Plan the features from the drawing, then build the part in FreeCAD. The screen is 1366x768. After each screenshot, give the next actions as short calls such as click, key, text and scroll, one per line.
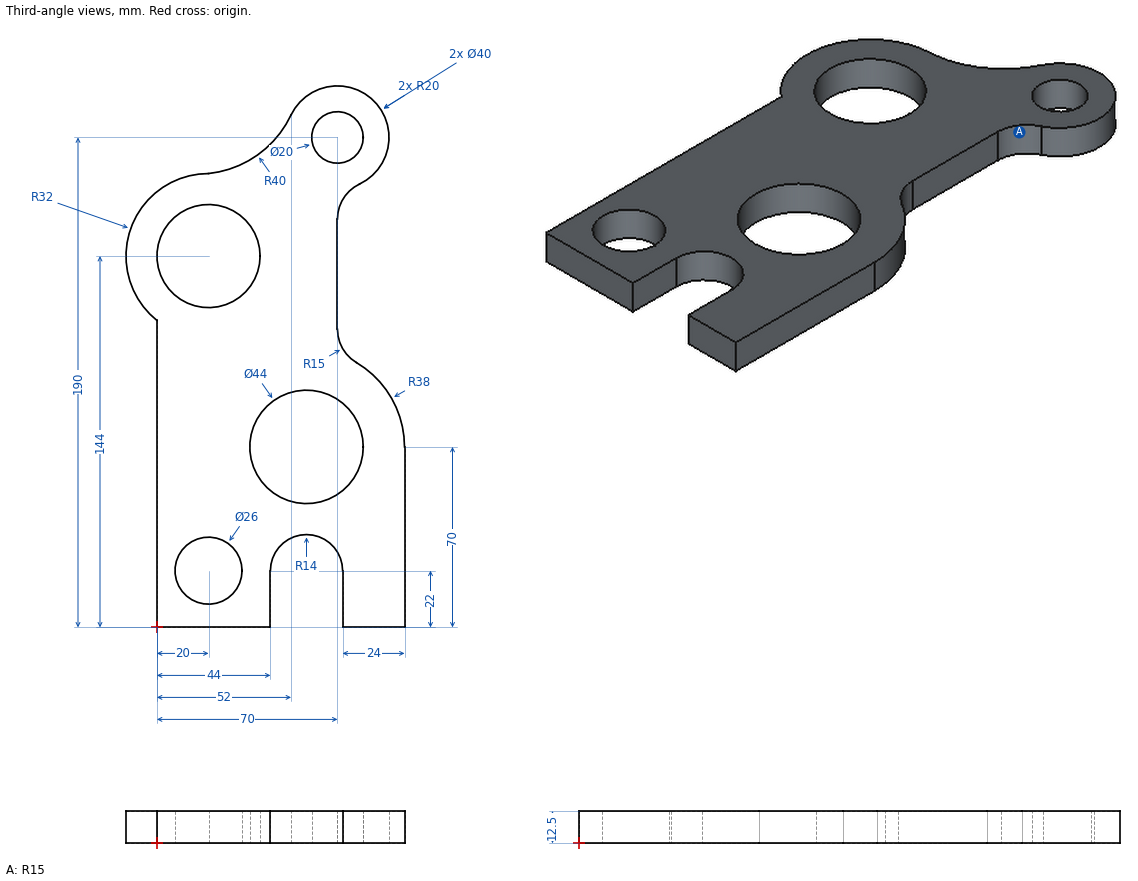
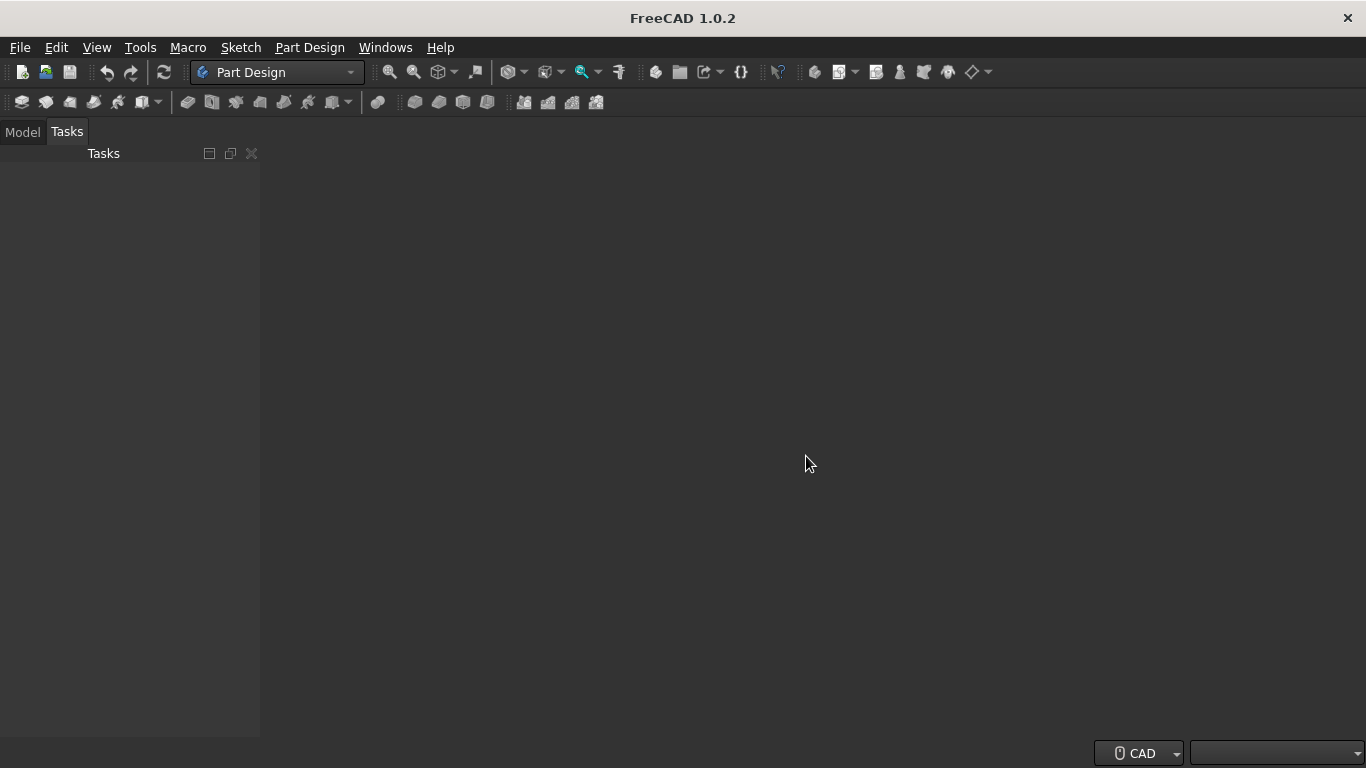
click(22, 72)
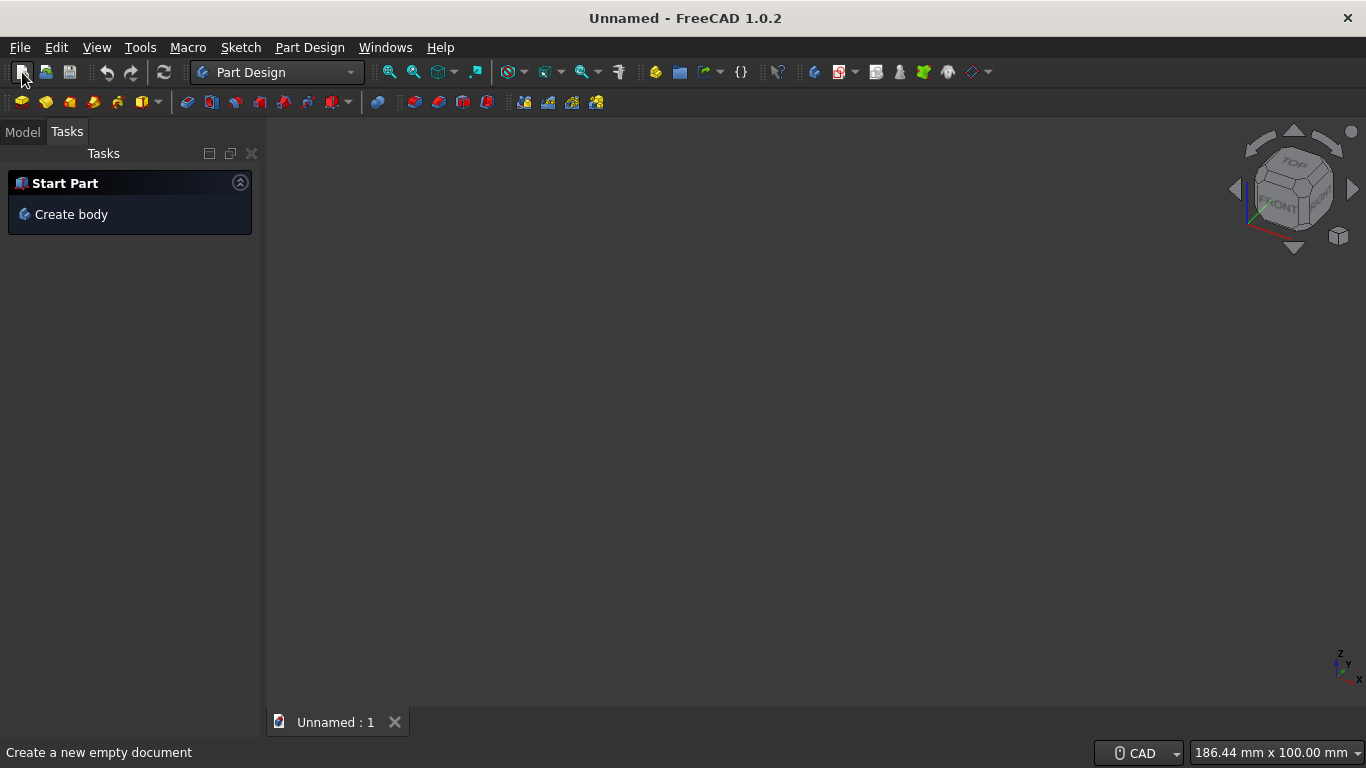
click(840, 72)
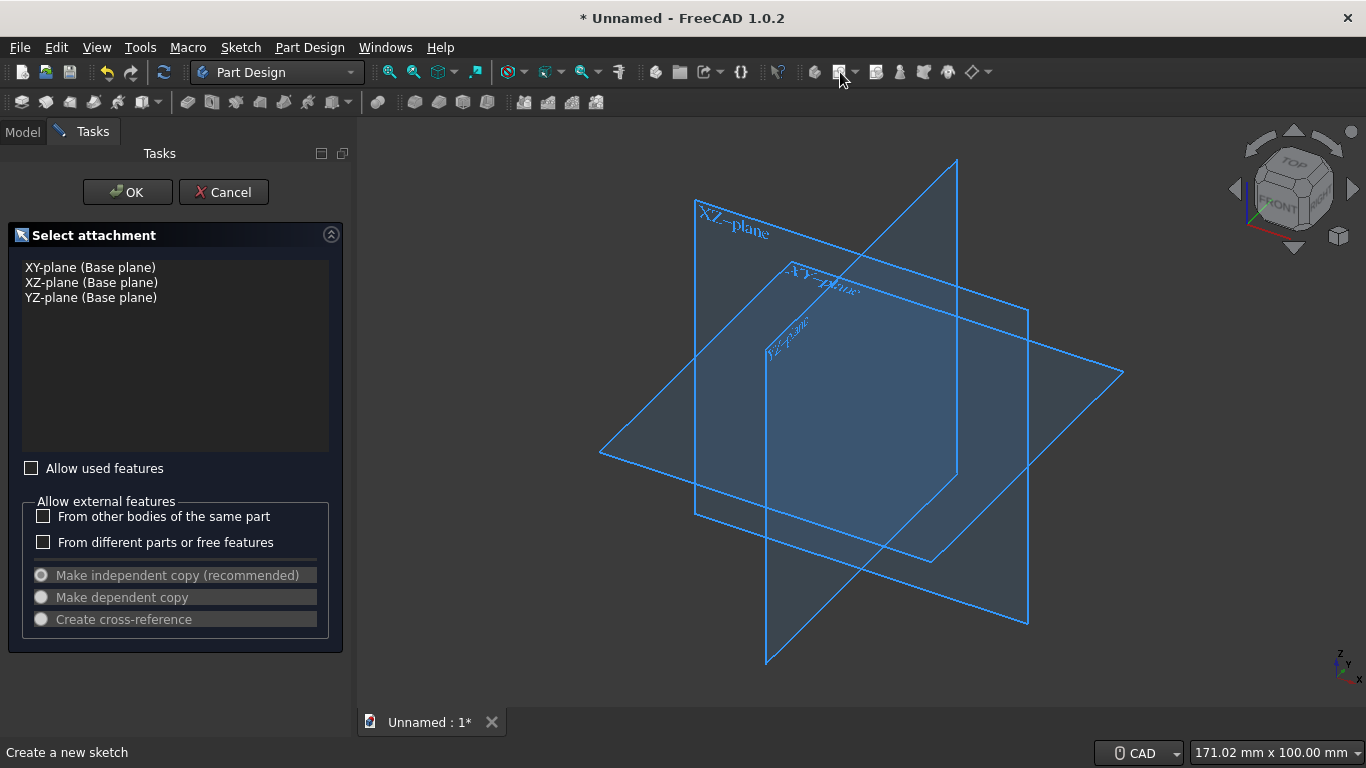
click(82, 268)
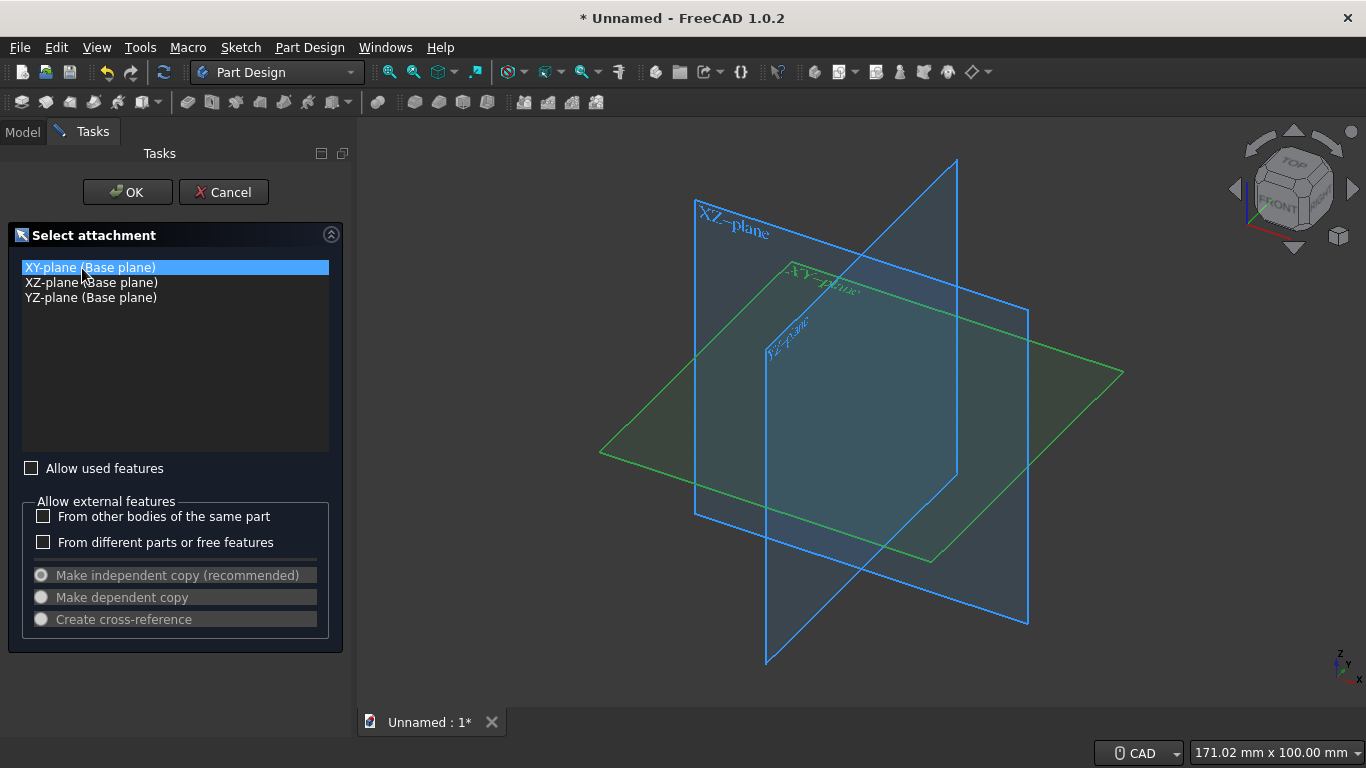
click(128, 192)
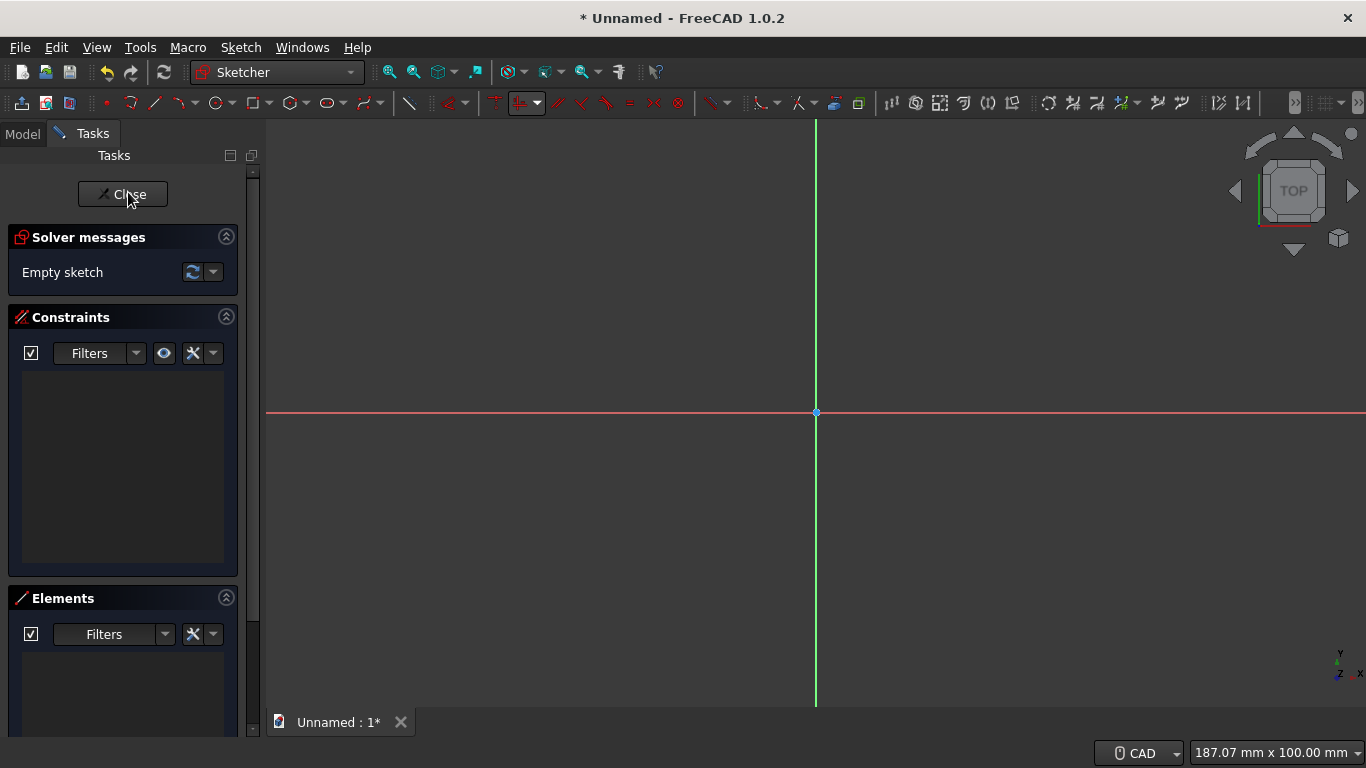
scroll(609, 667, down, 6)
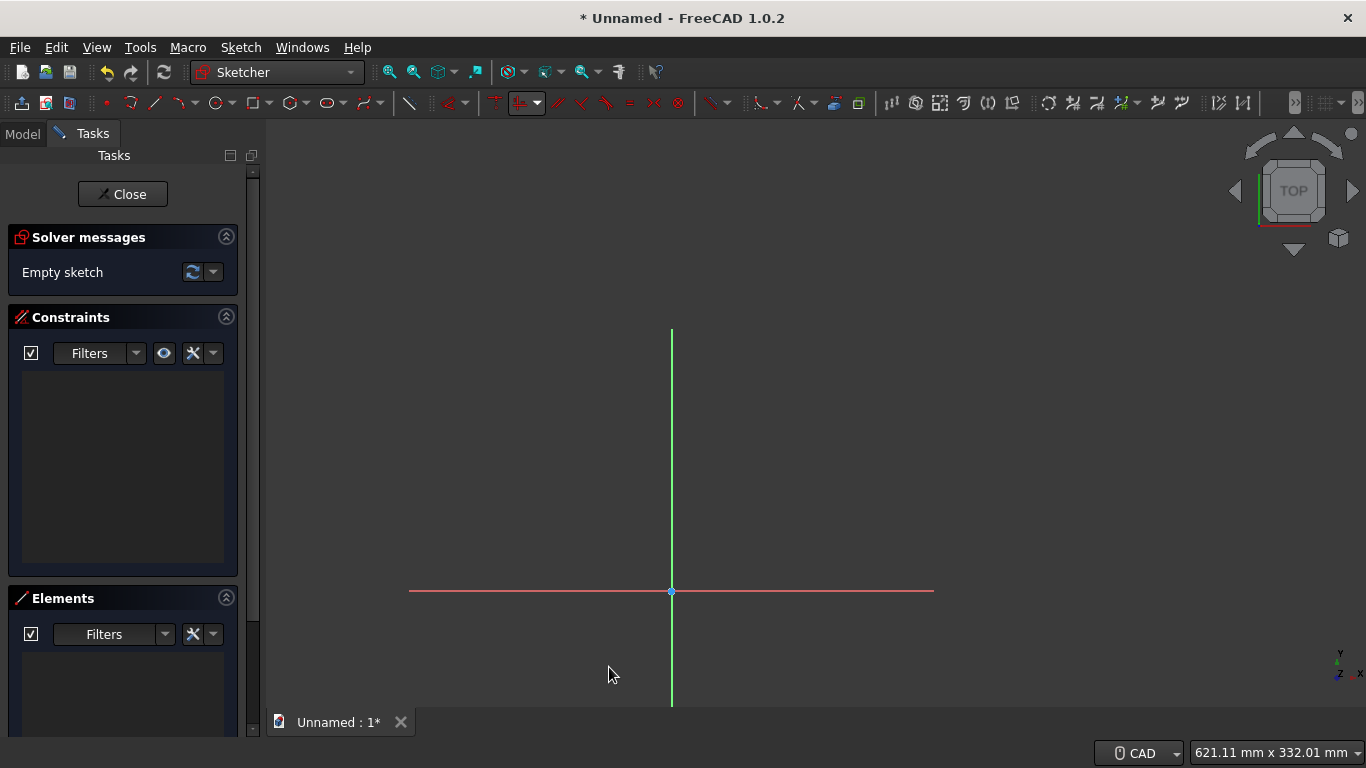
click(132, 104)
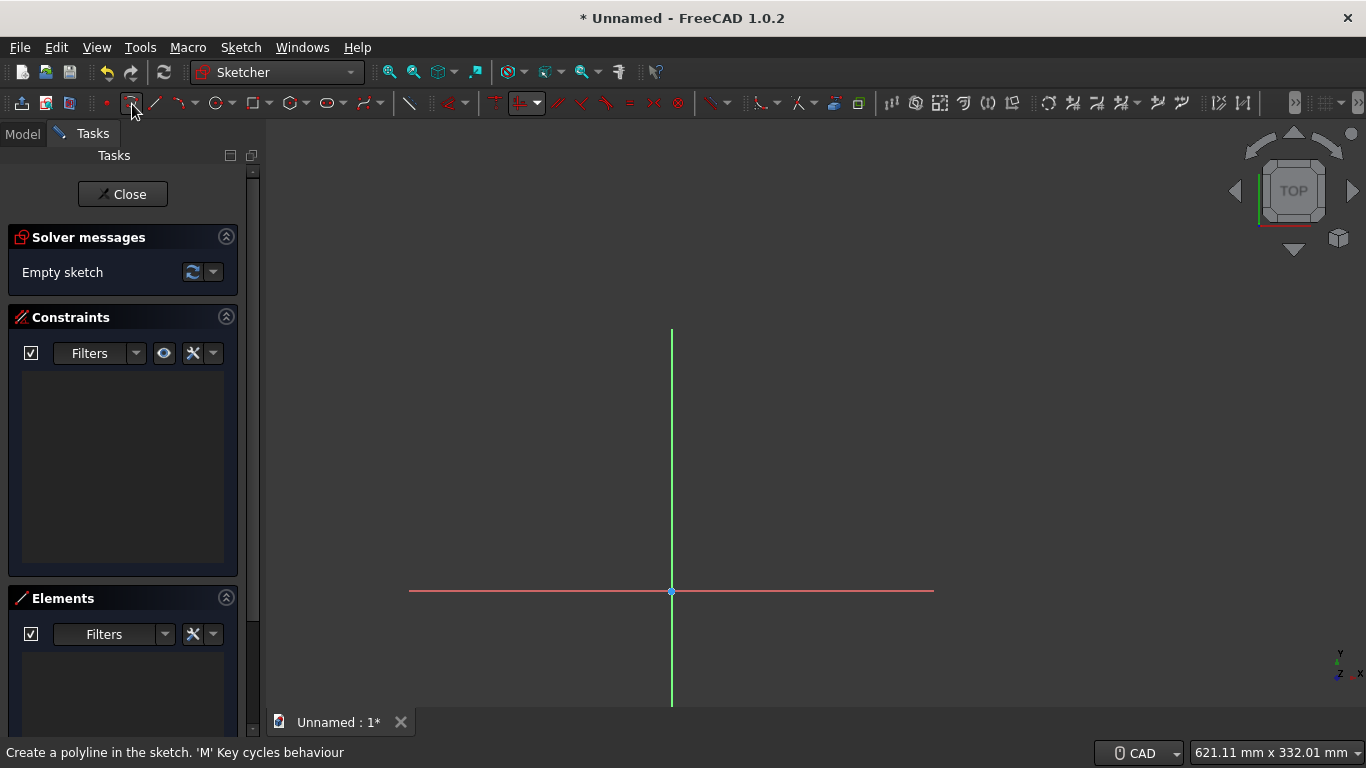
click(672, 380)
click(672, 591)
click(749, 582)
click(749, 552)
right_click(749, 552)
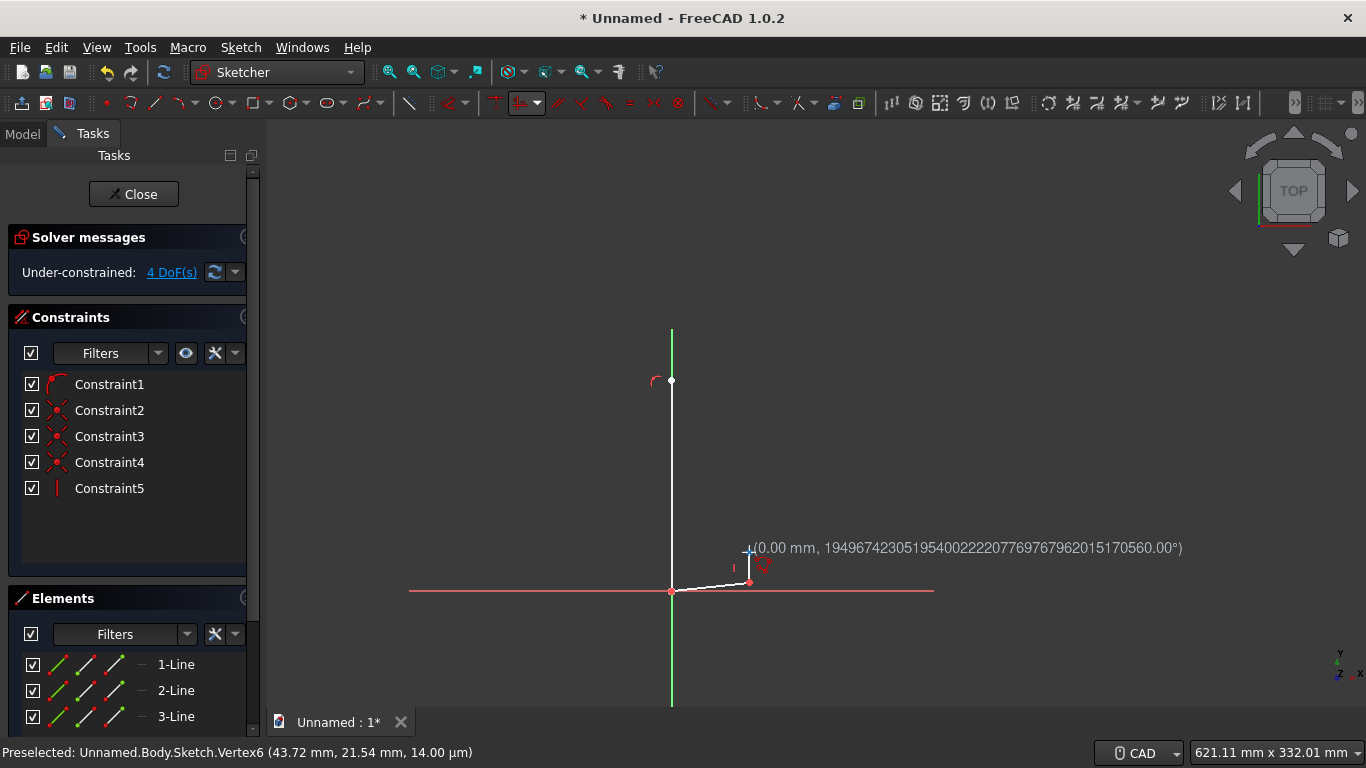
click(799, 552)
click(799, 591)
click(842, 582)
click(842, 467)
right_click(842, 467)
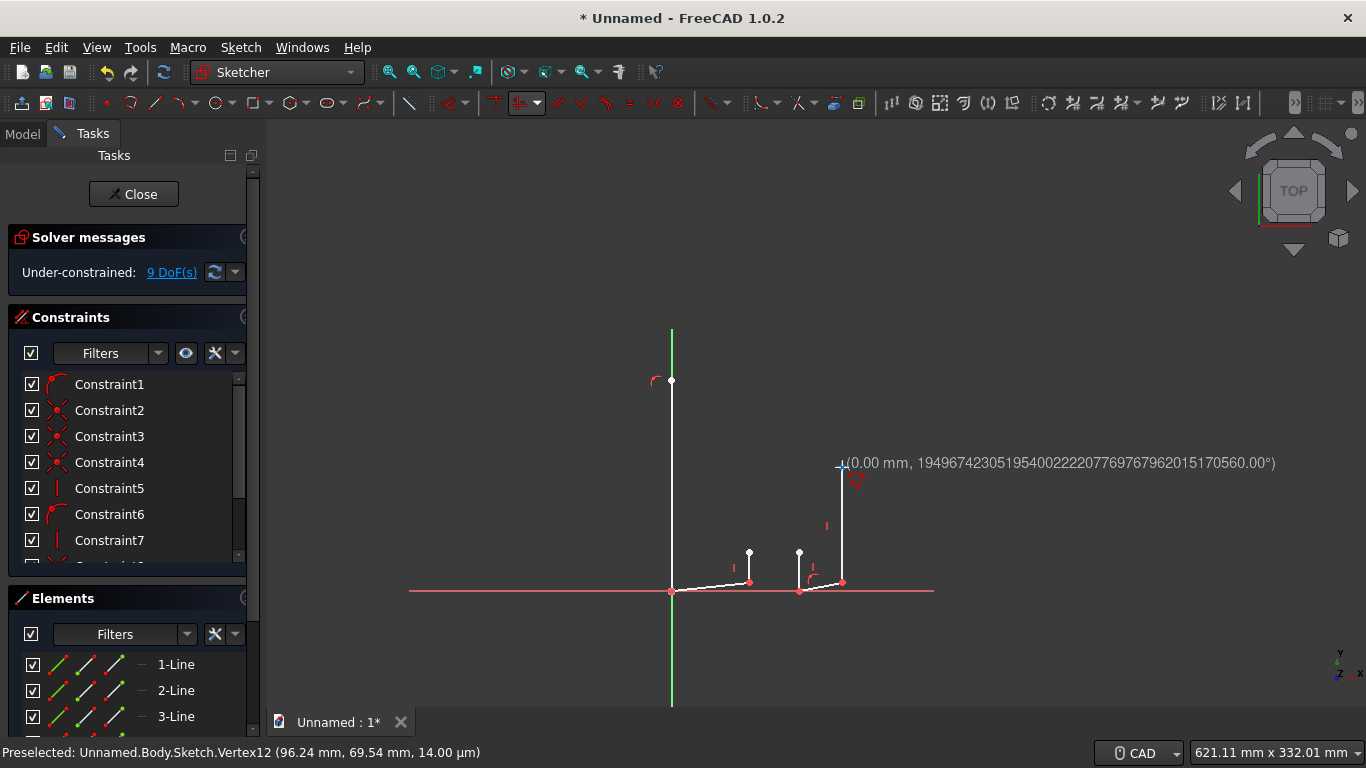
click(156, 104)